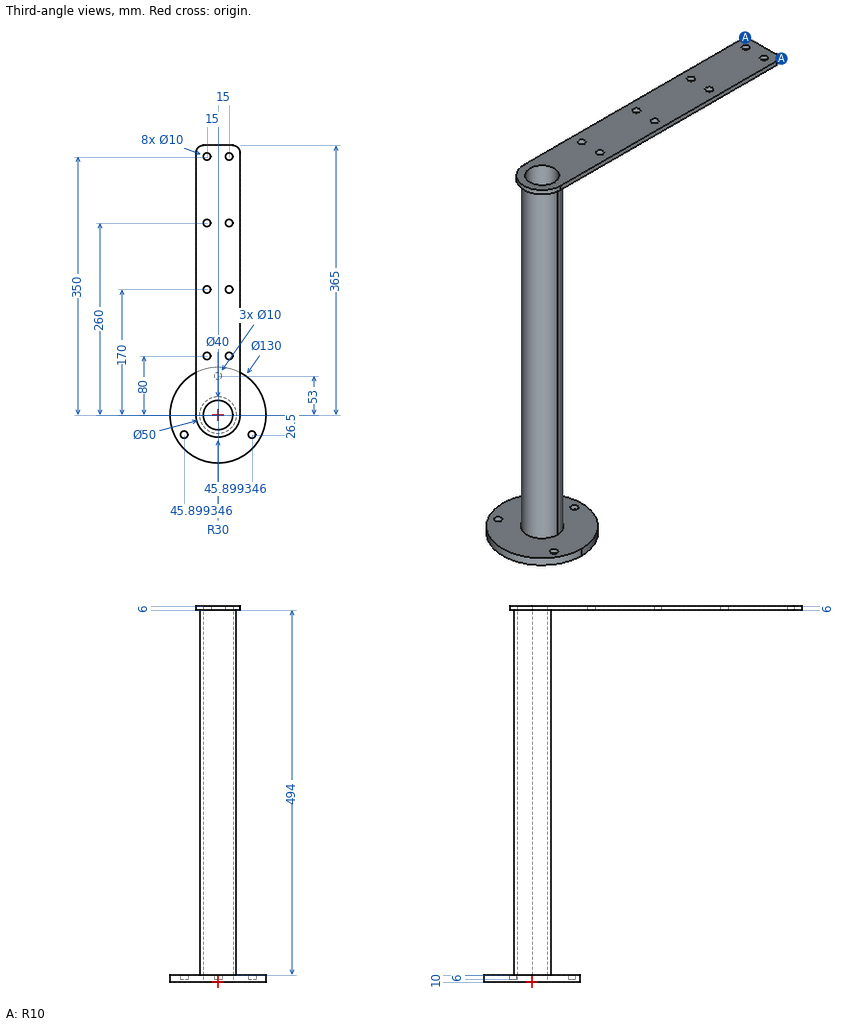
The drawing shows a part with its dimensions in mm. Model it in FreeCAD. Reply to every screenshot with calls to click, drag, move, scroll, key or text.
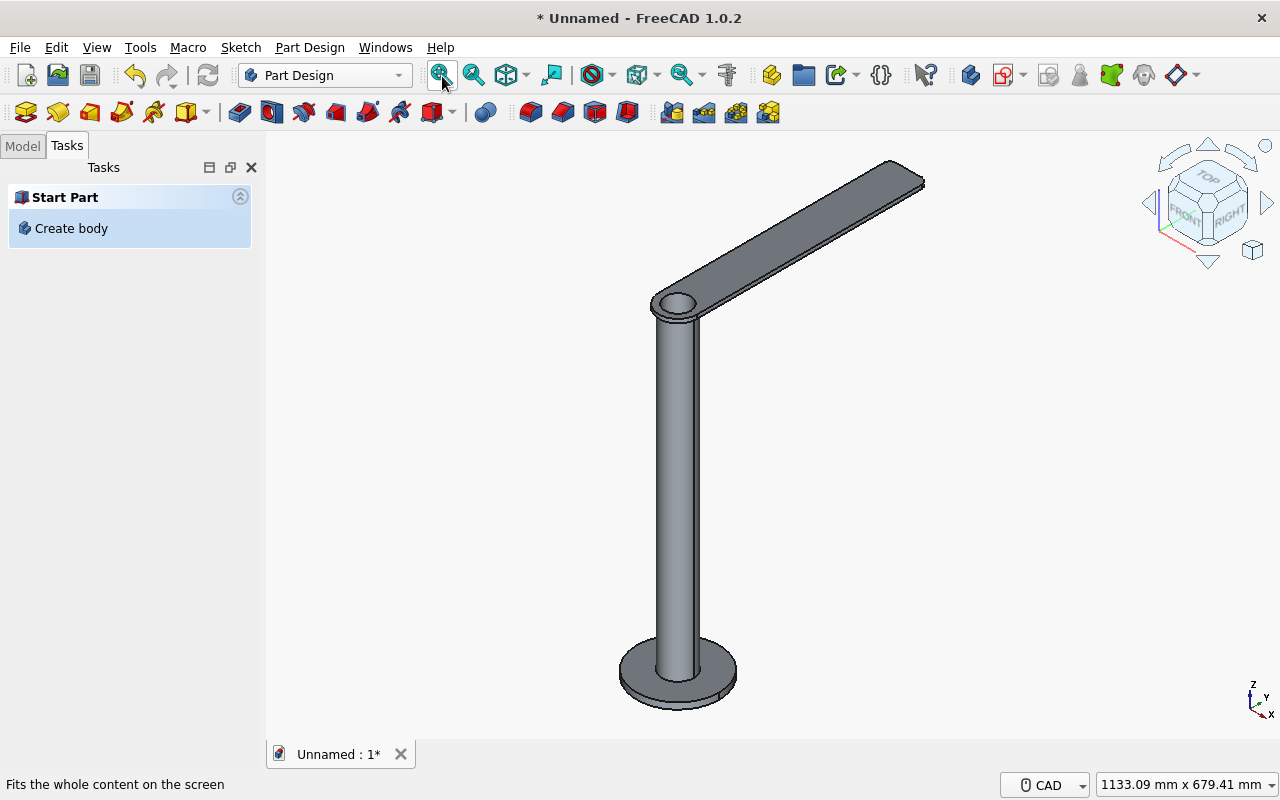
click(855, 200)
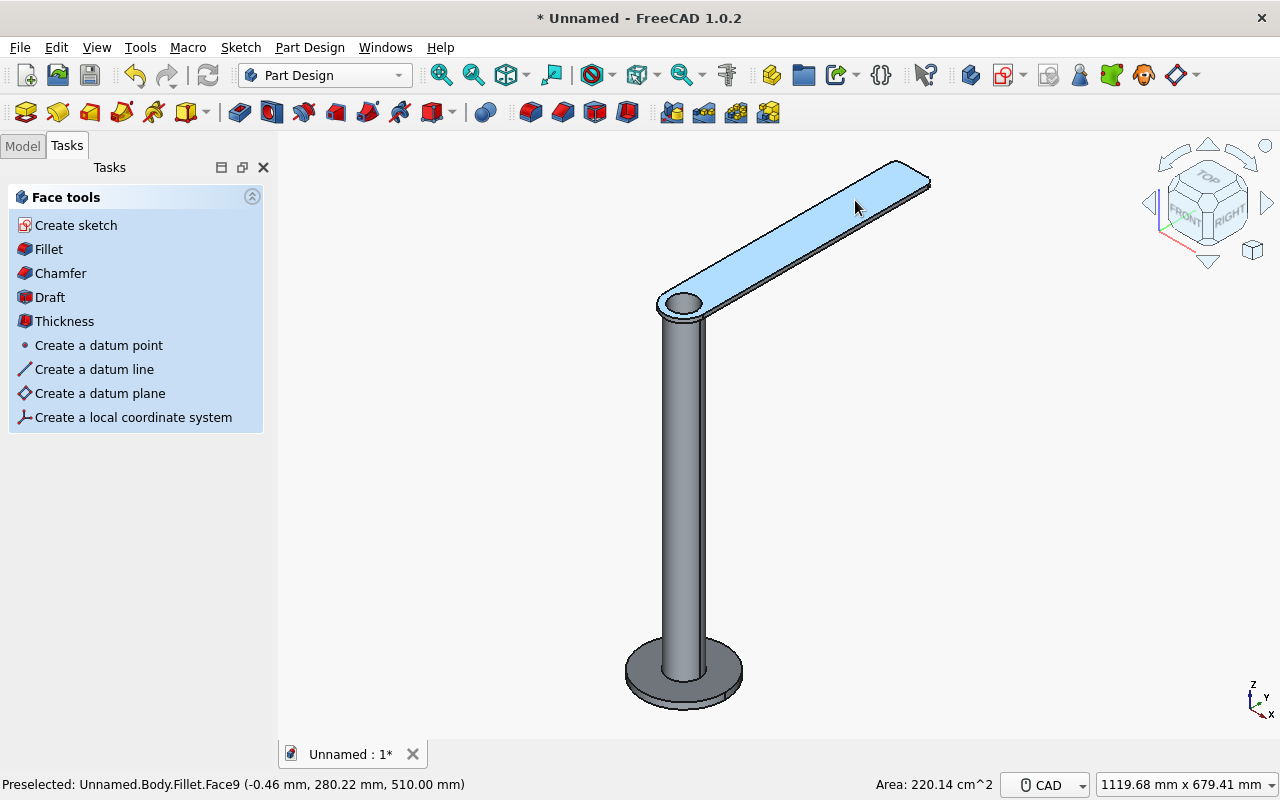
click(1004, 76)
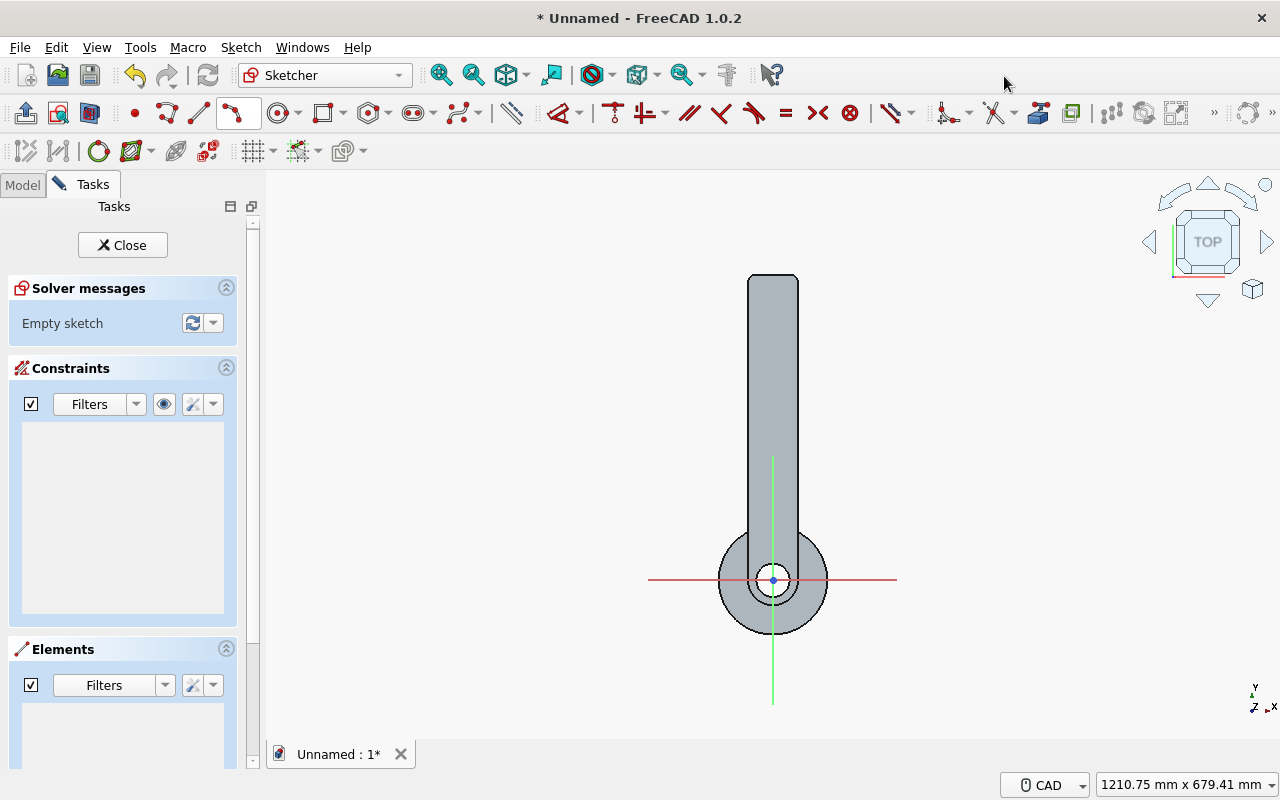
click(278, 114)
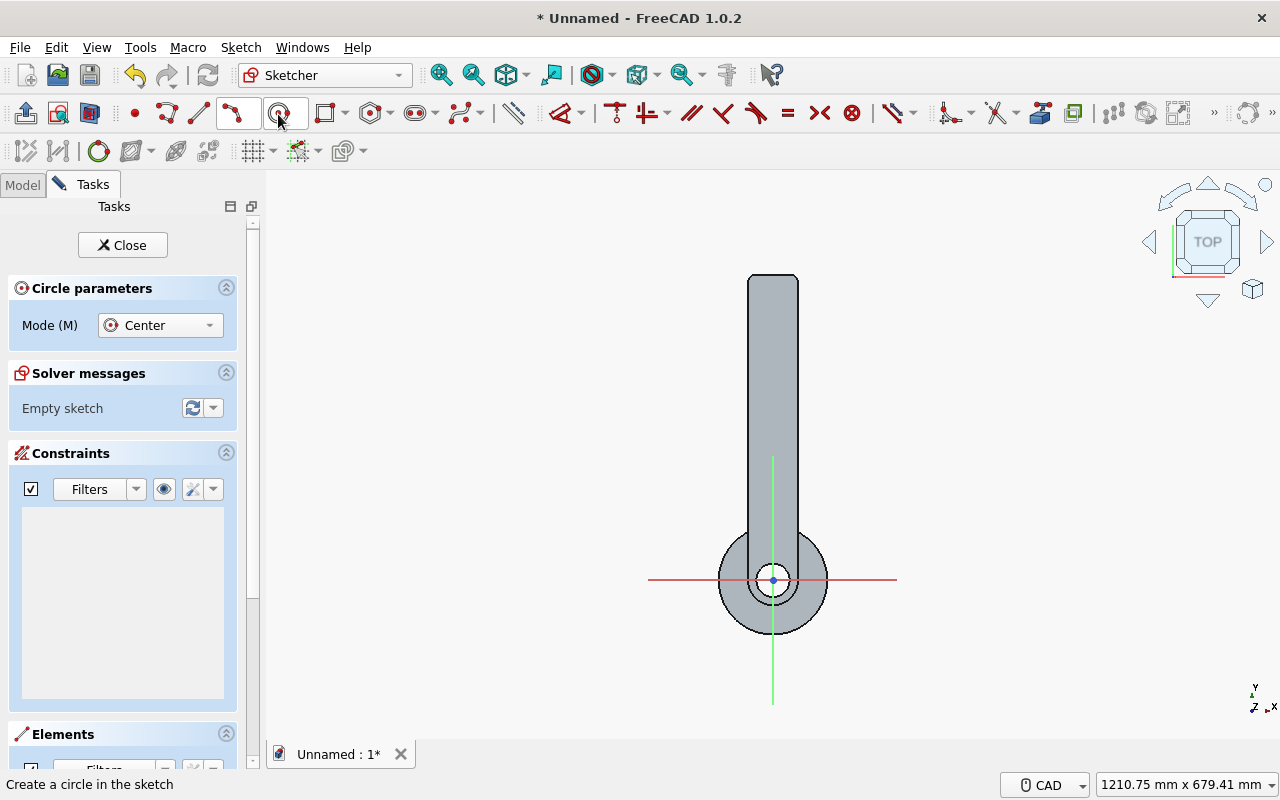
scroll(760, 287, up, 9)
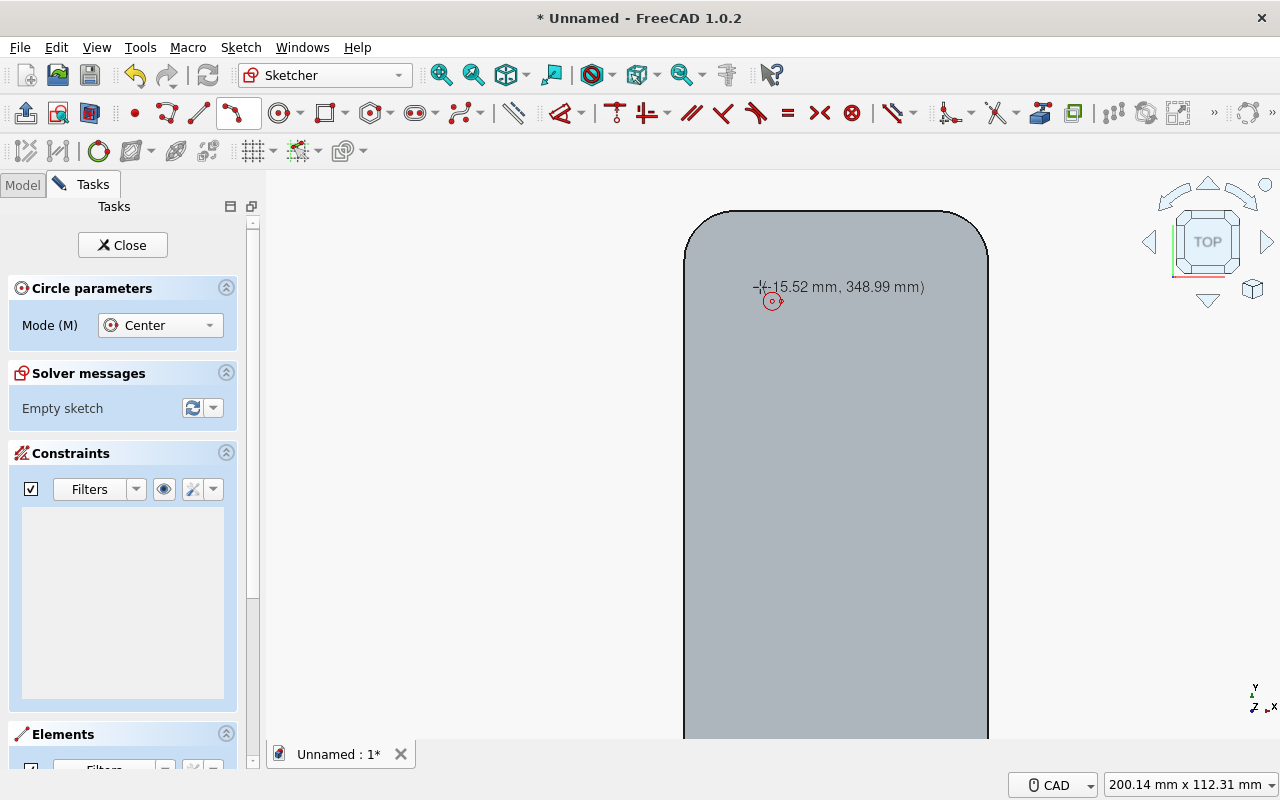
scroll(671, 276, down, 8)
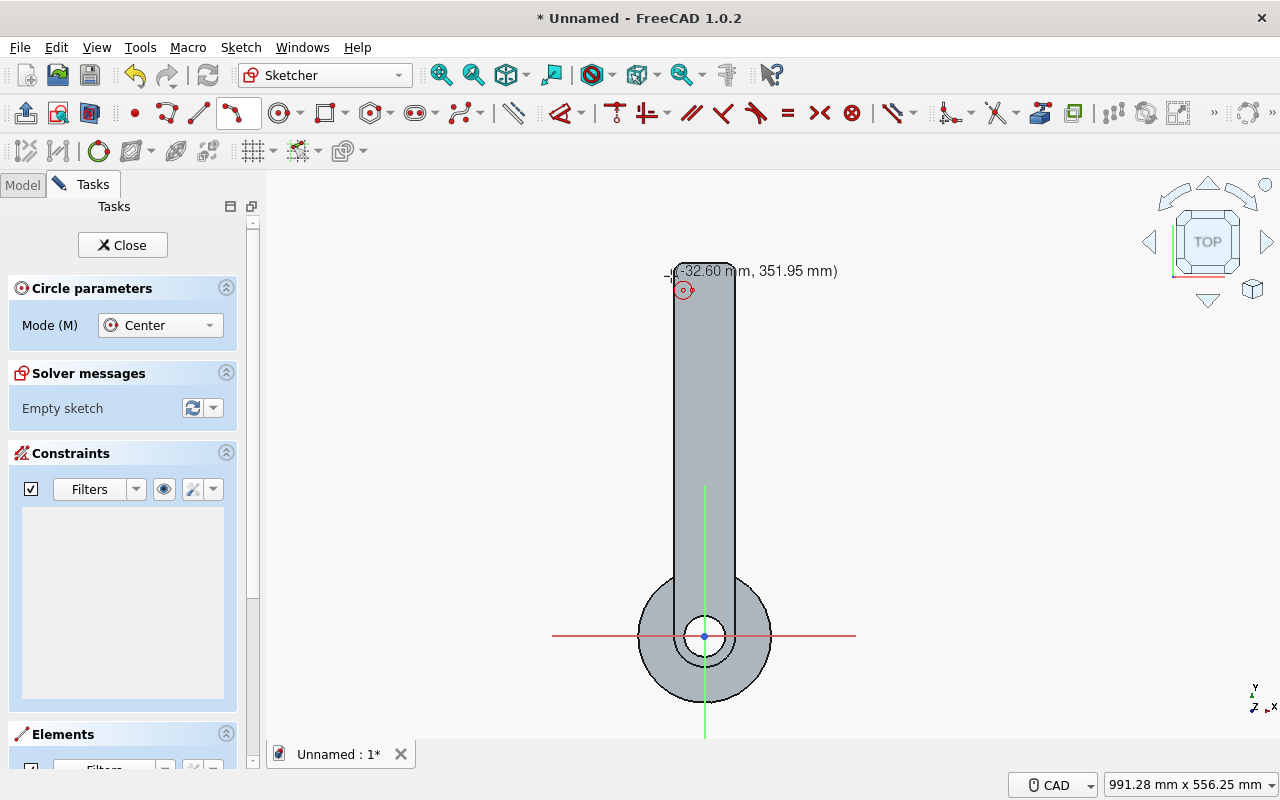
click(689, 278)
move(686, 275)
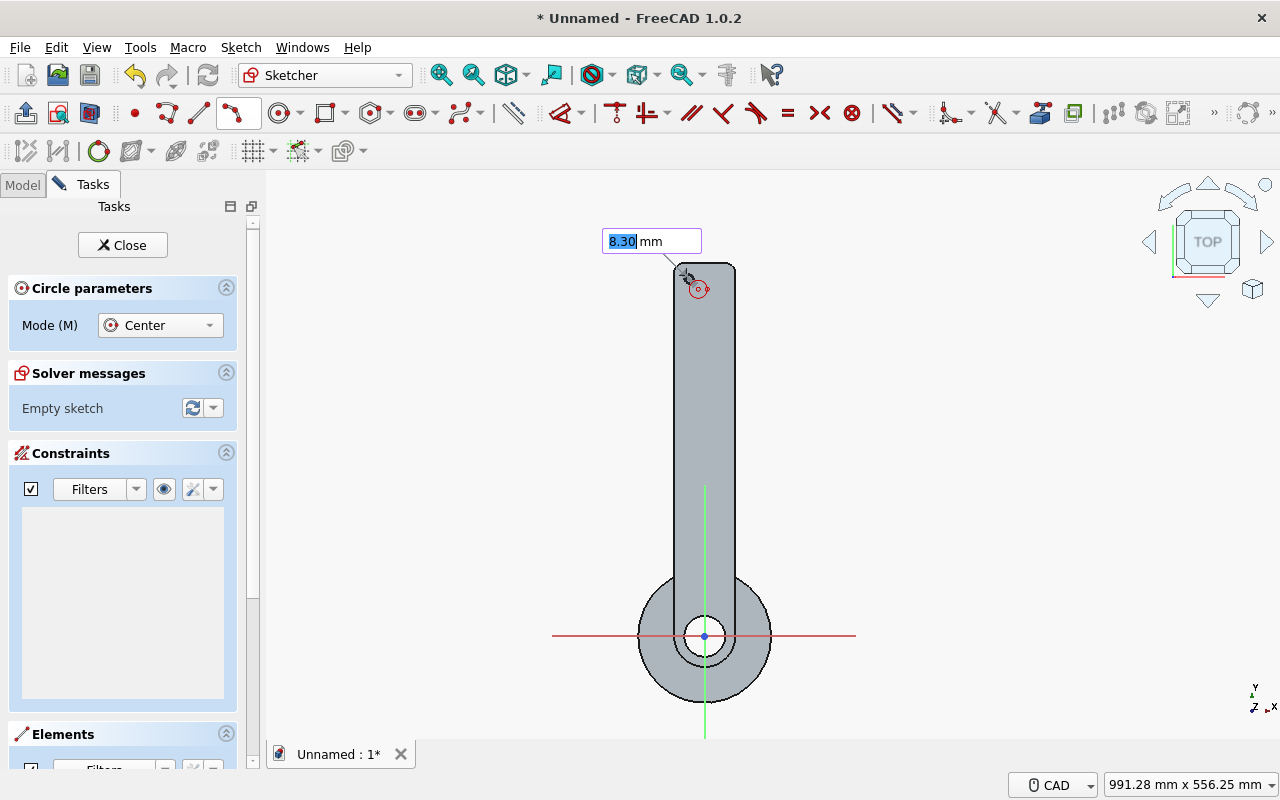
text(10)
key(Return)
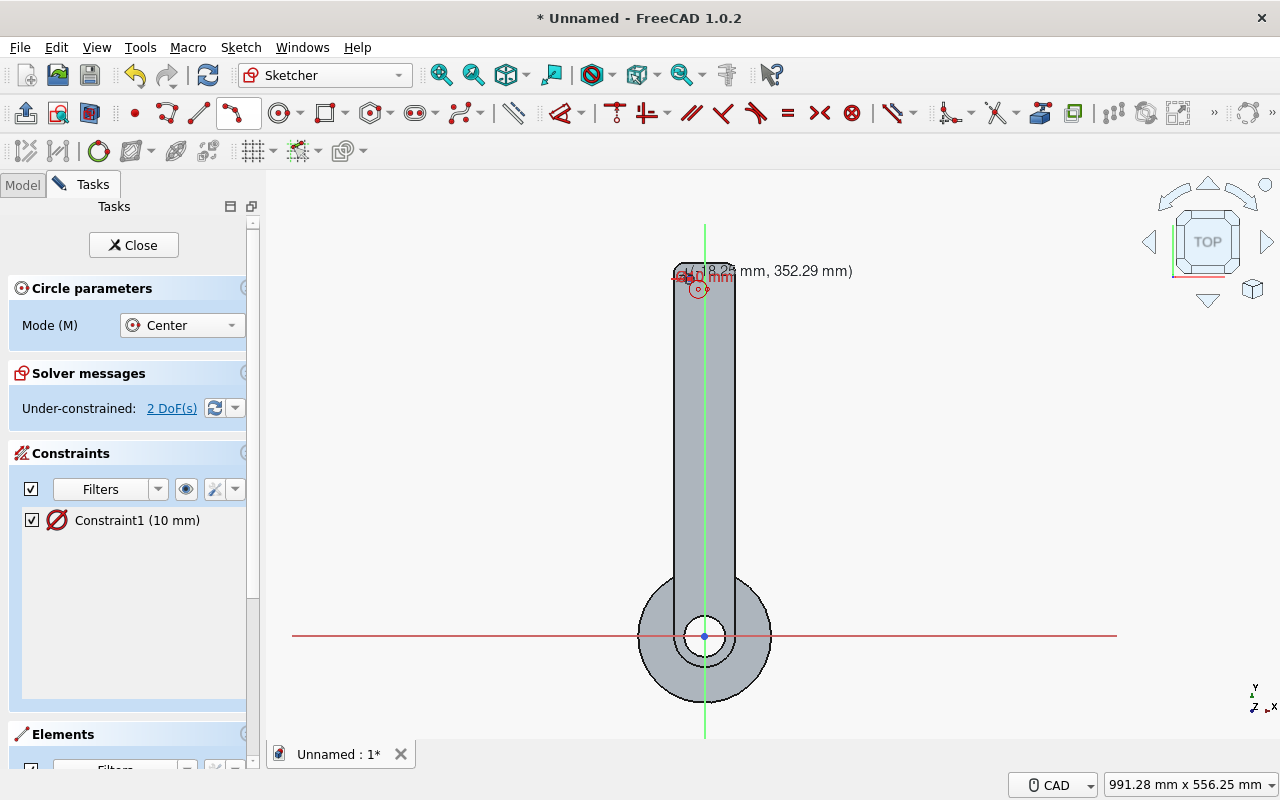
scroll(720, 278, up, 8)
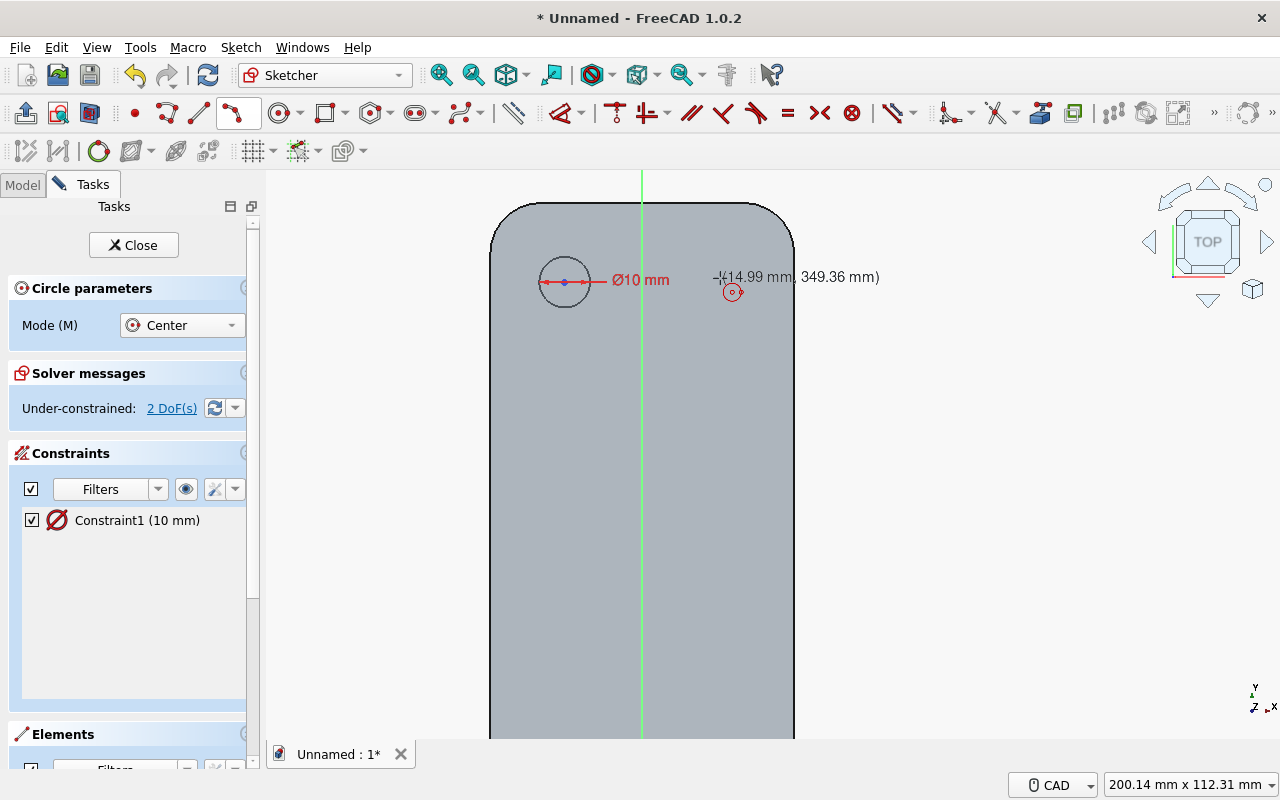
scroll(720, 278, down, 8)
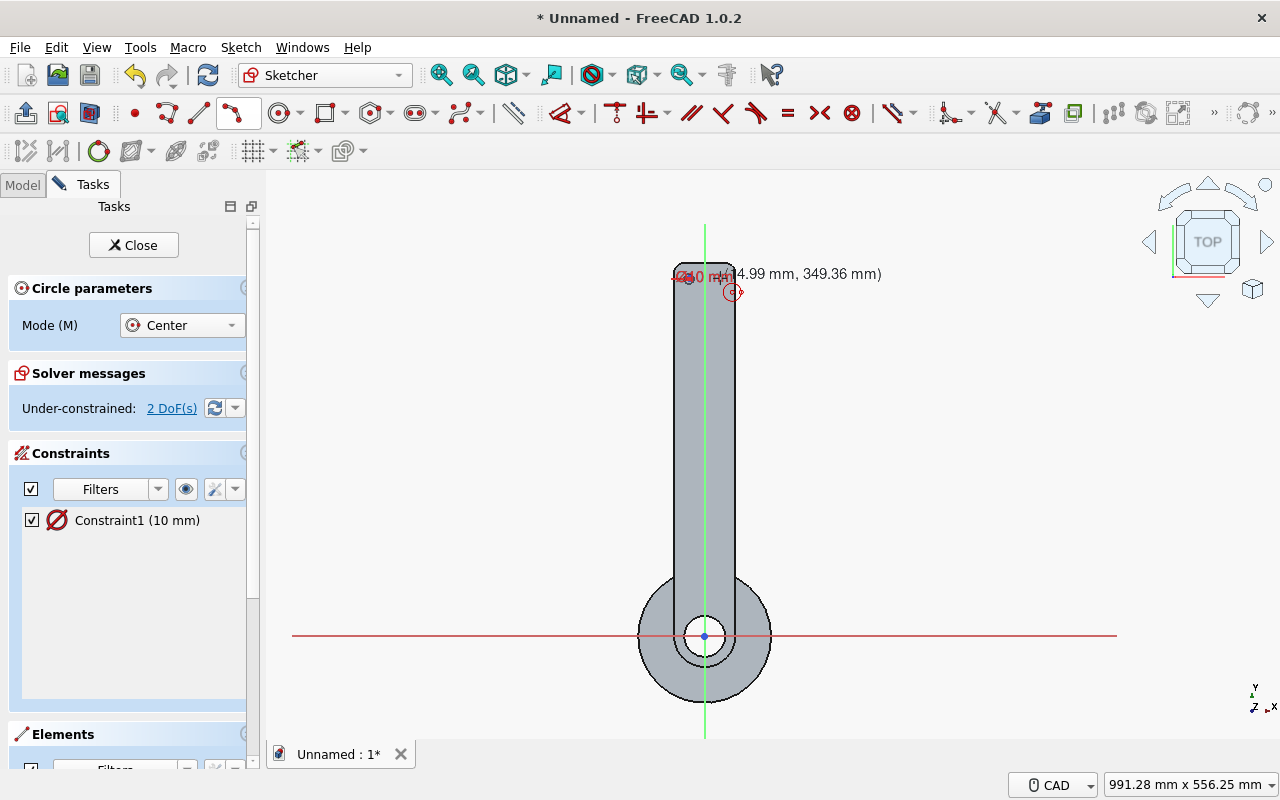
click(720, 278)
move(724, 275)